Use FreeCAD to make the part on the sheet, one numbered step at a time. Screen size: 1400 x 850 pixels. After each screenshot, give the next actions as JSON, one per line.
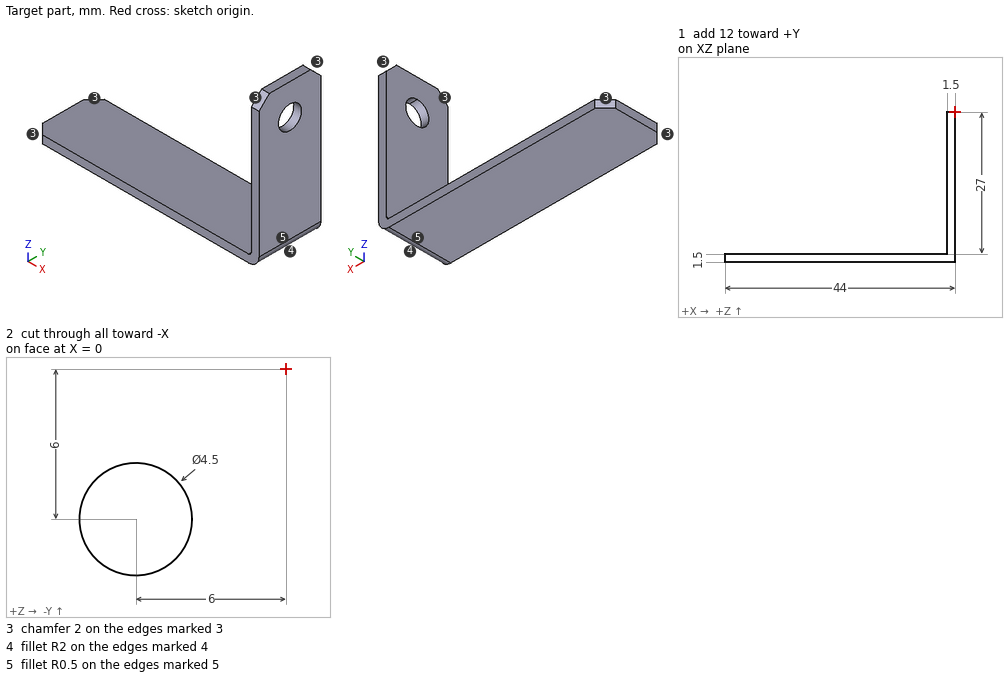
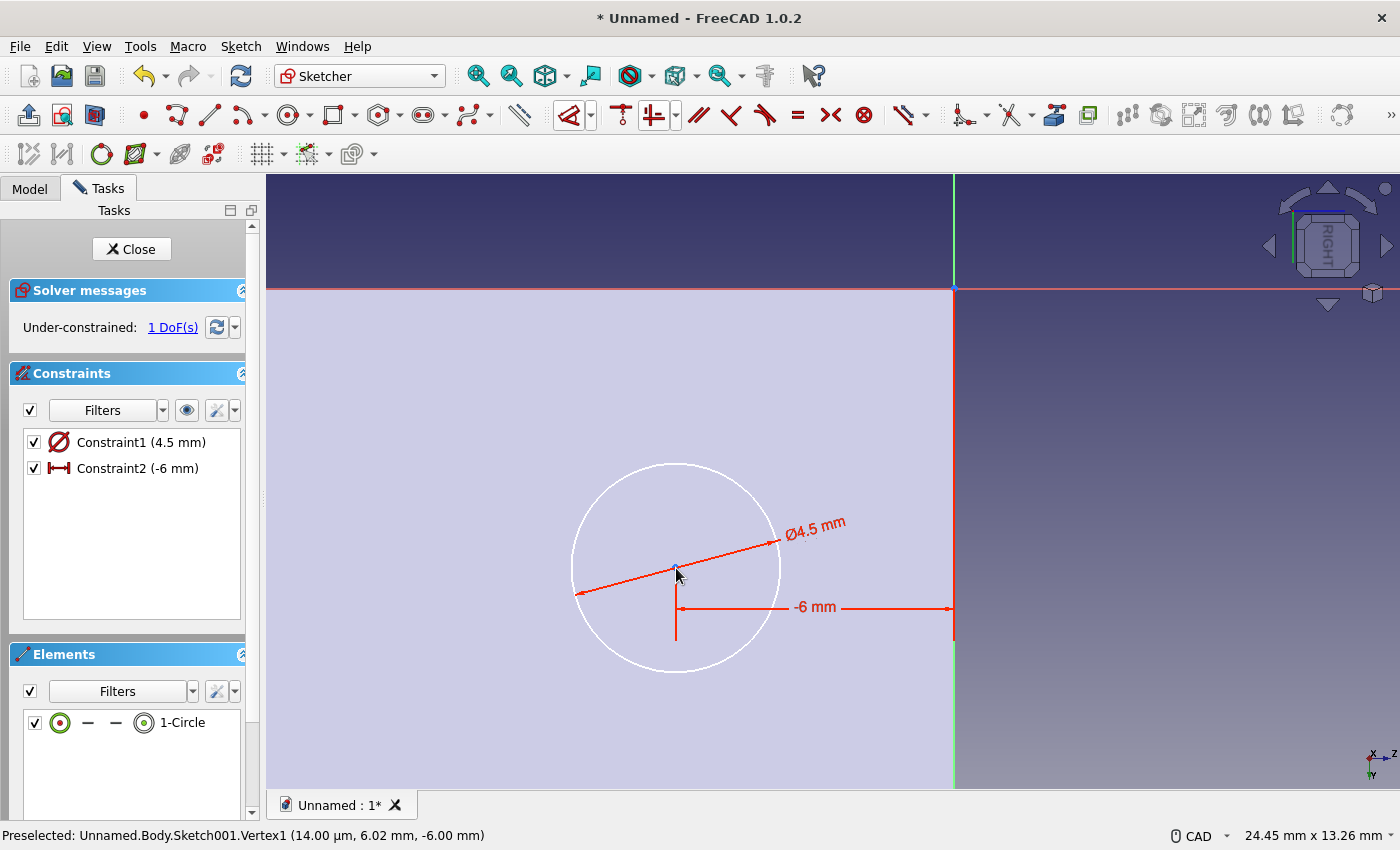
{"action": "left_click", "coordinate": [676, 568]}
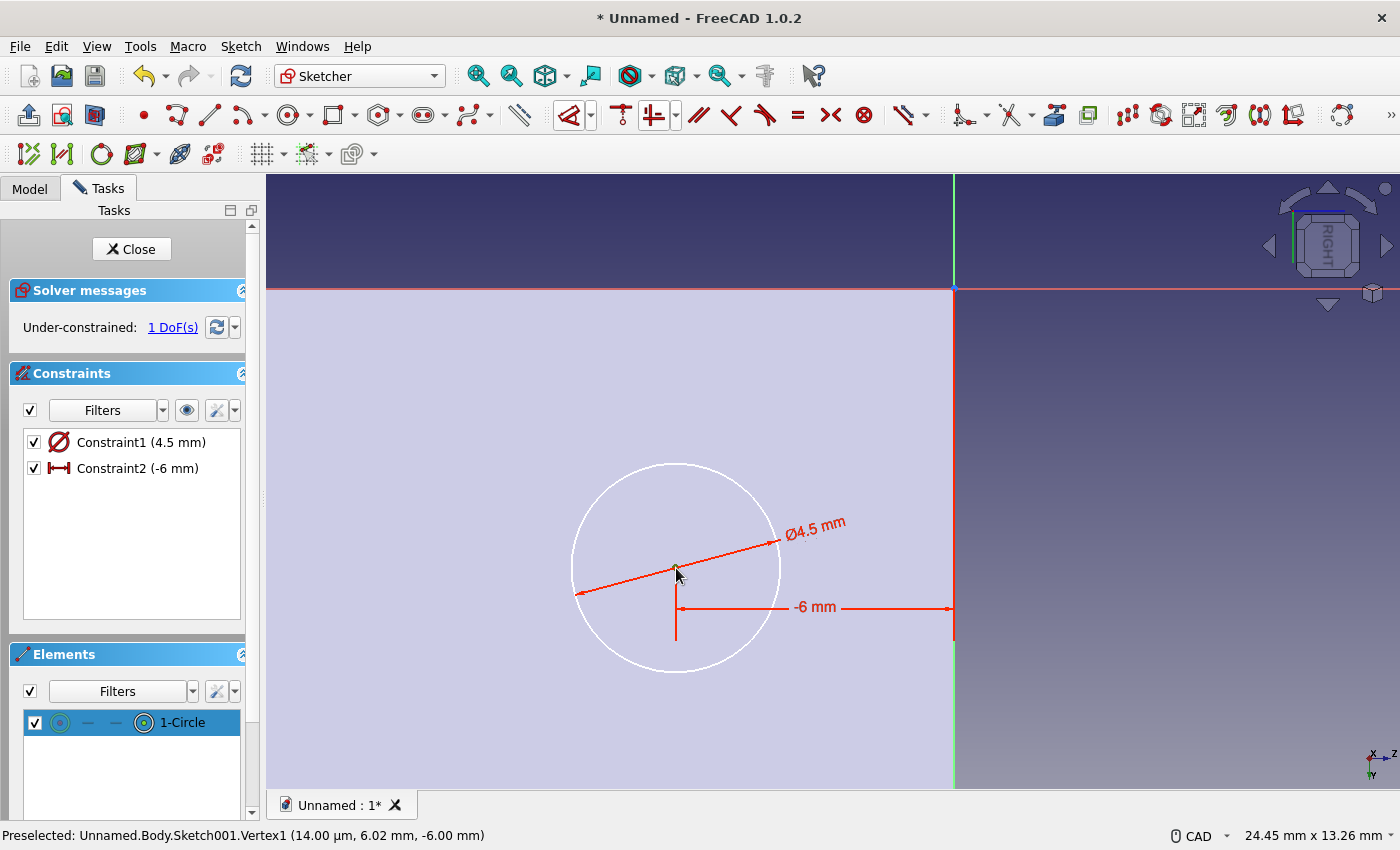
{"action": "key", "text": "i"}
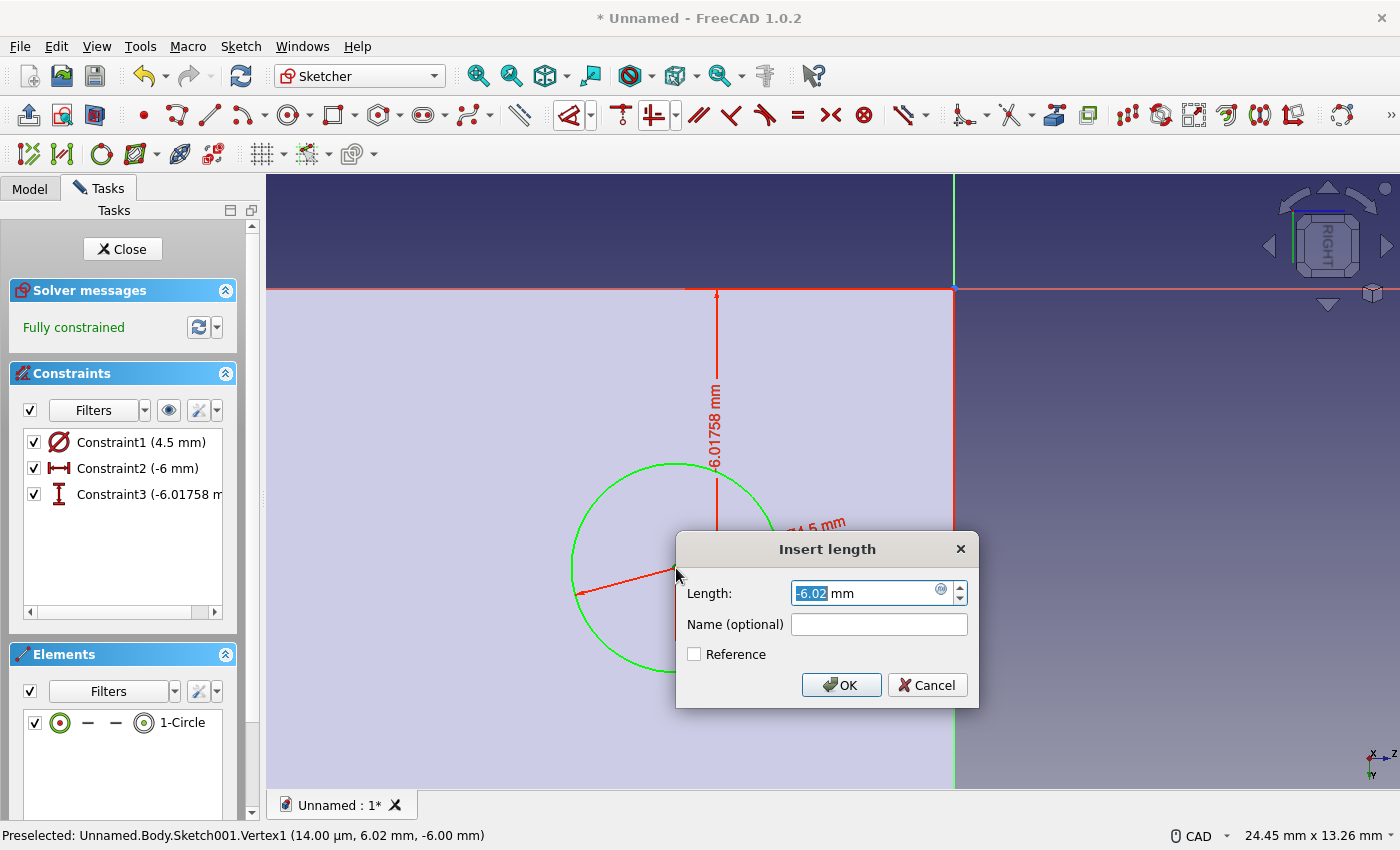
{"action": "type", "text": "-6"}
{"action": "key", "text": "Return"}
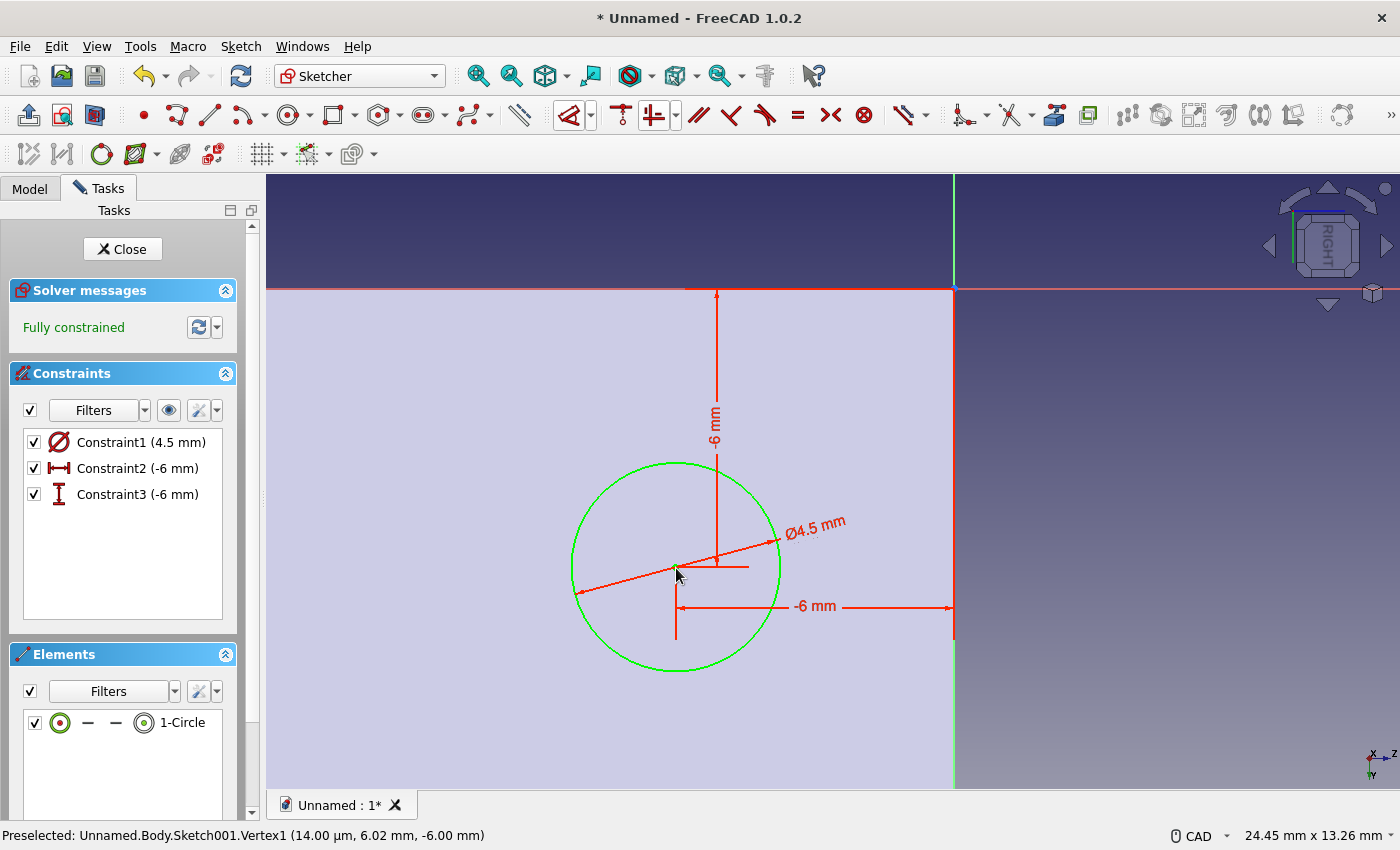
{"action": "left_click", "coordinate": [123, 249]}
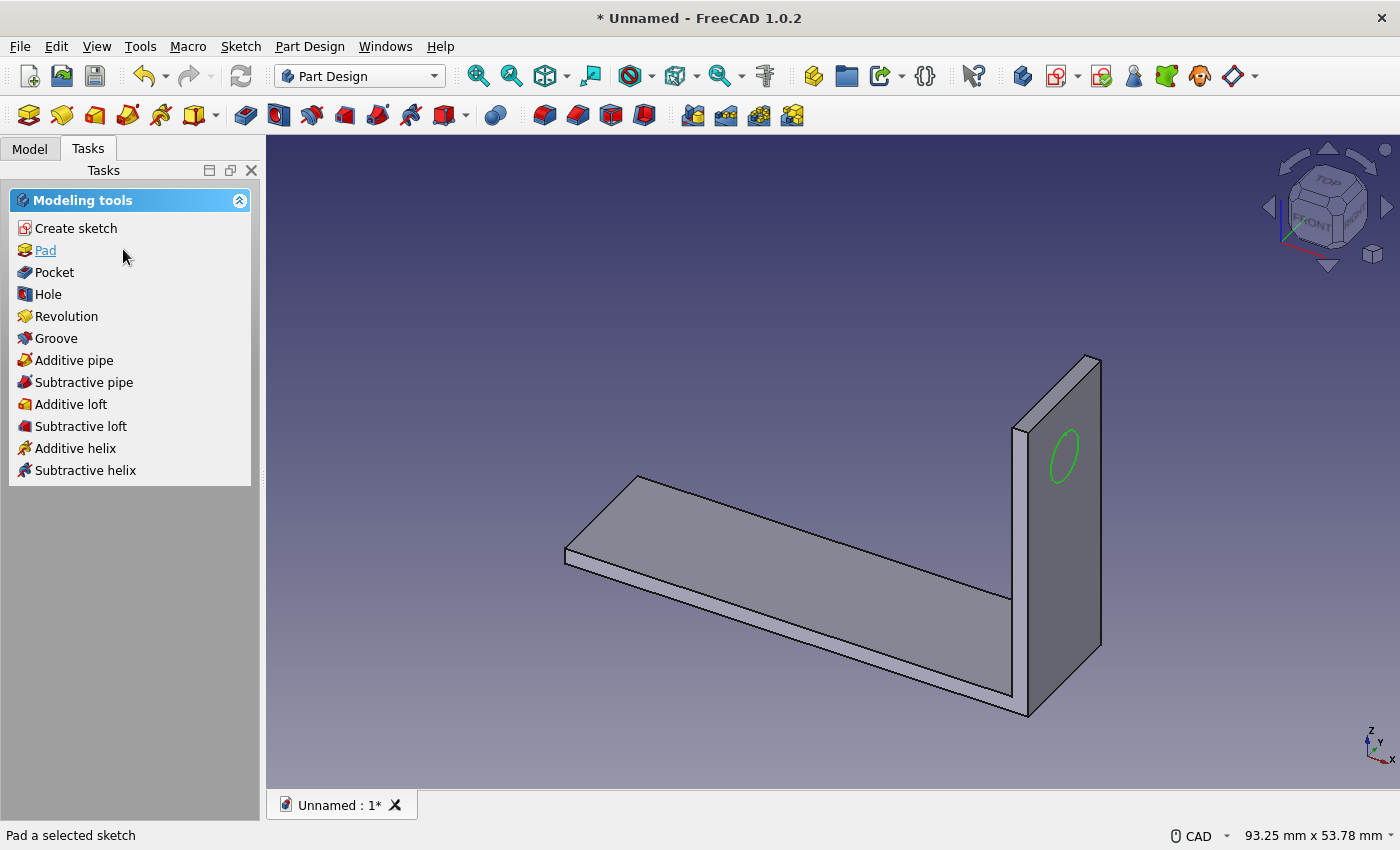
{"action": "left_click", "coordinate": [246, 116]}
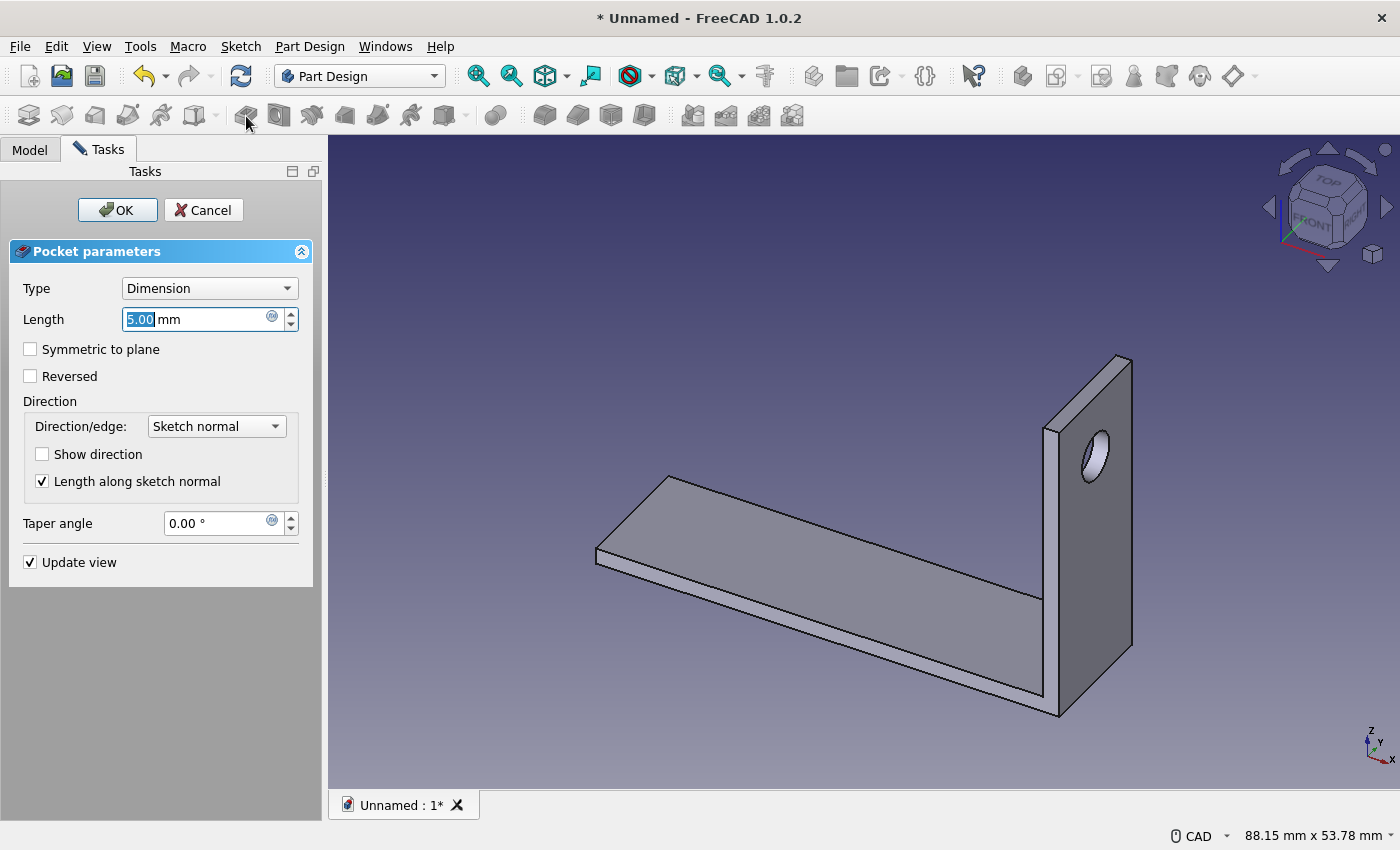
{"action": "left_click", "coordinate": [210, 288]}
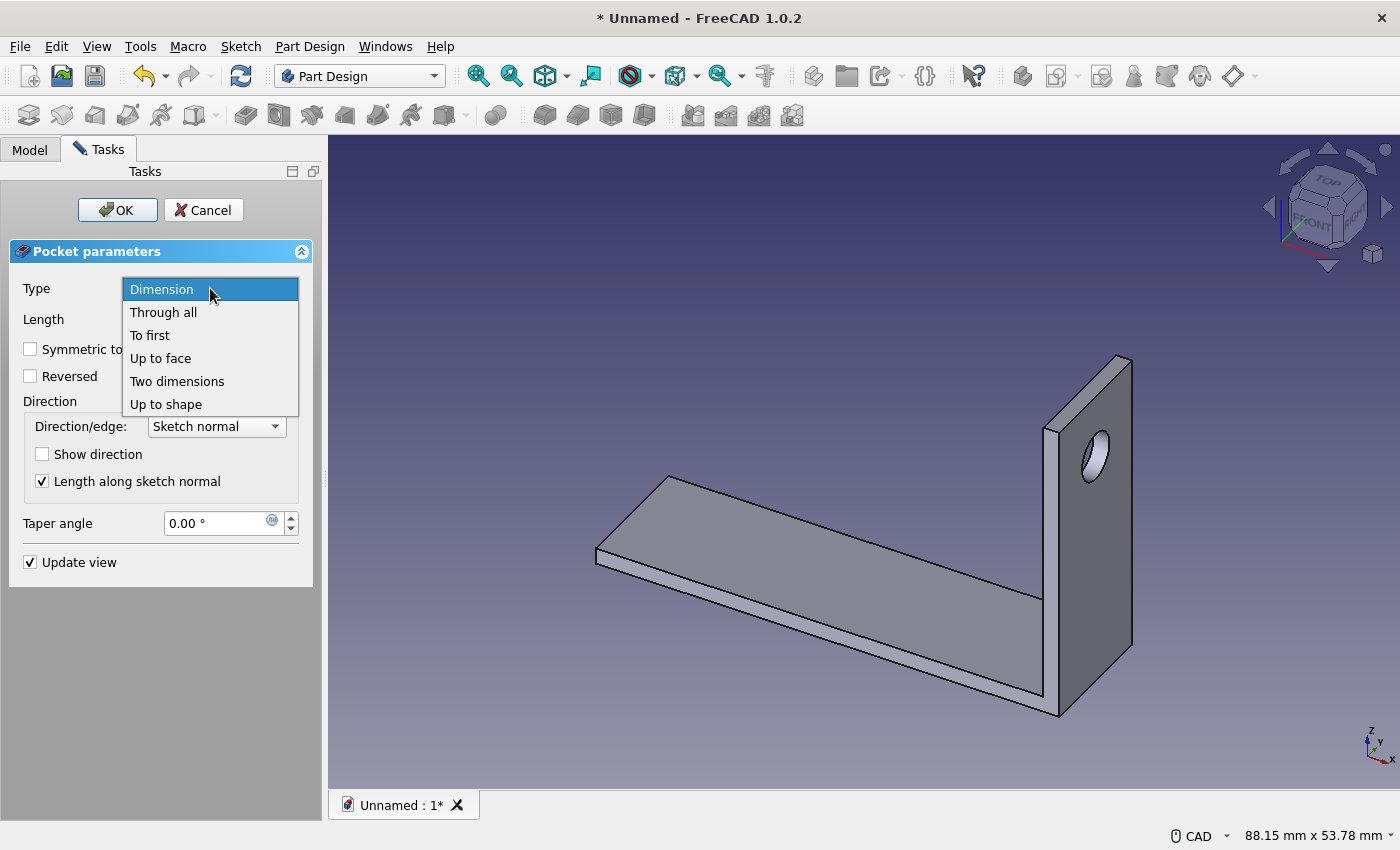
{"action": "left_click", "coordinate": [208, 312]}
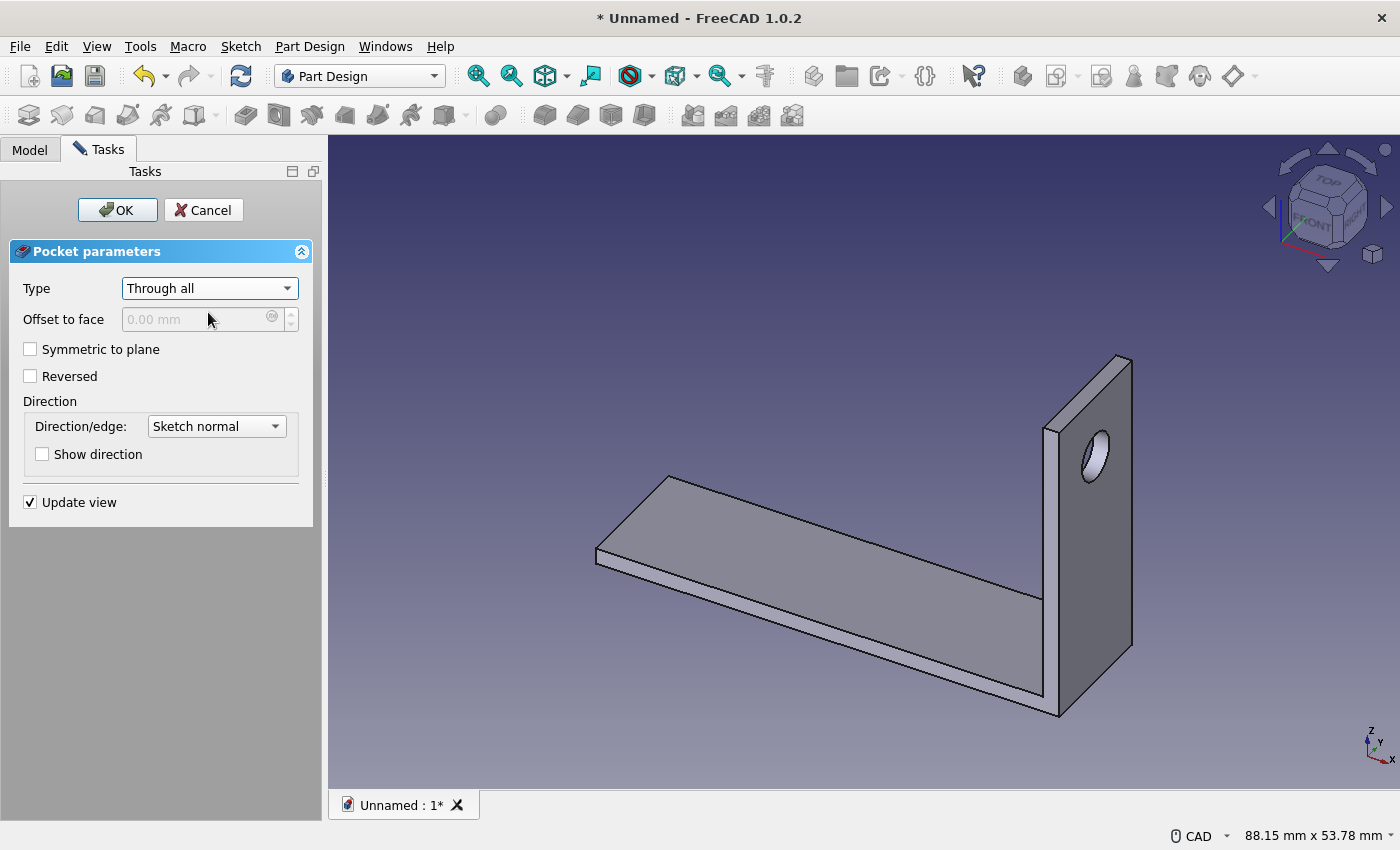
{"action": "left_click", "coordinate": [118, 210]}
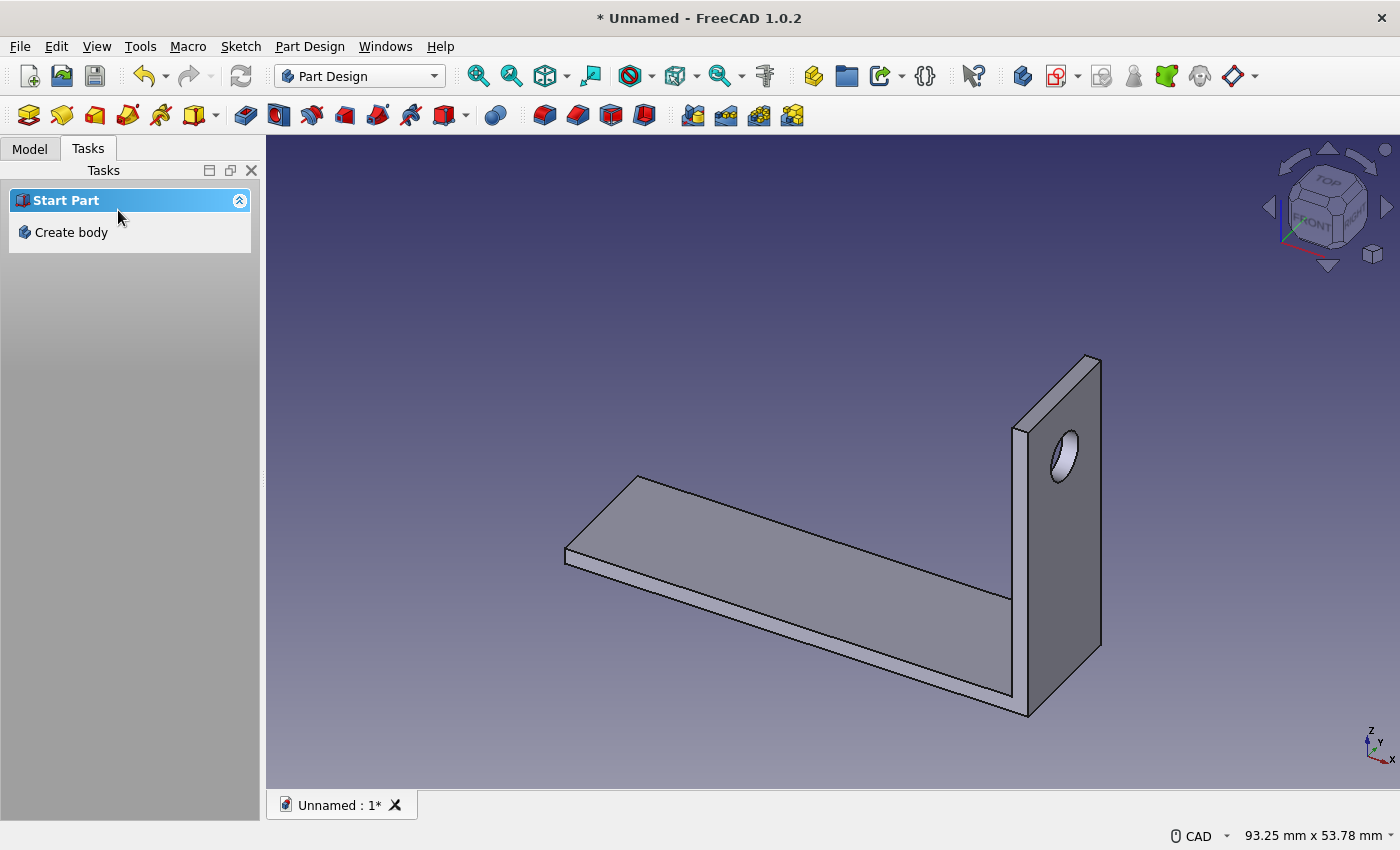
{"action": "left_click", "coordinate": [1020, 429]}